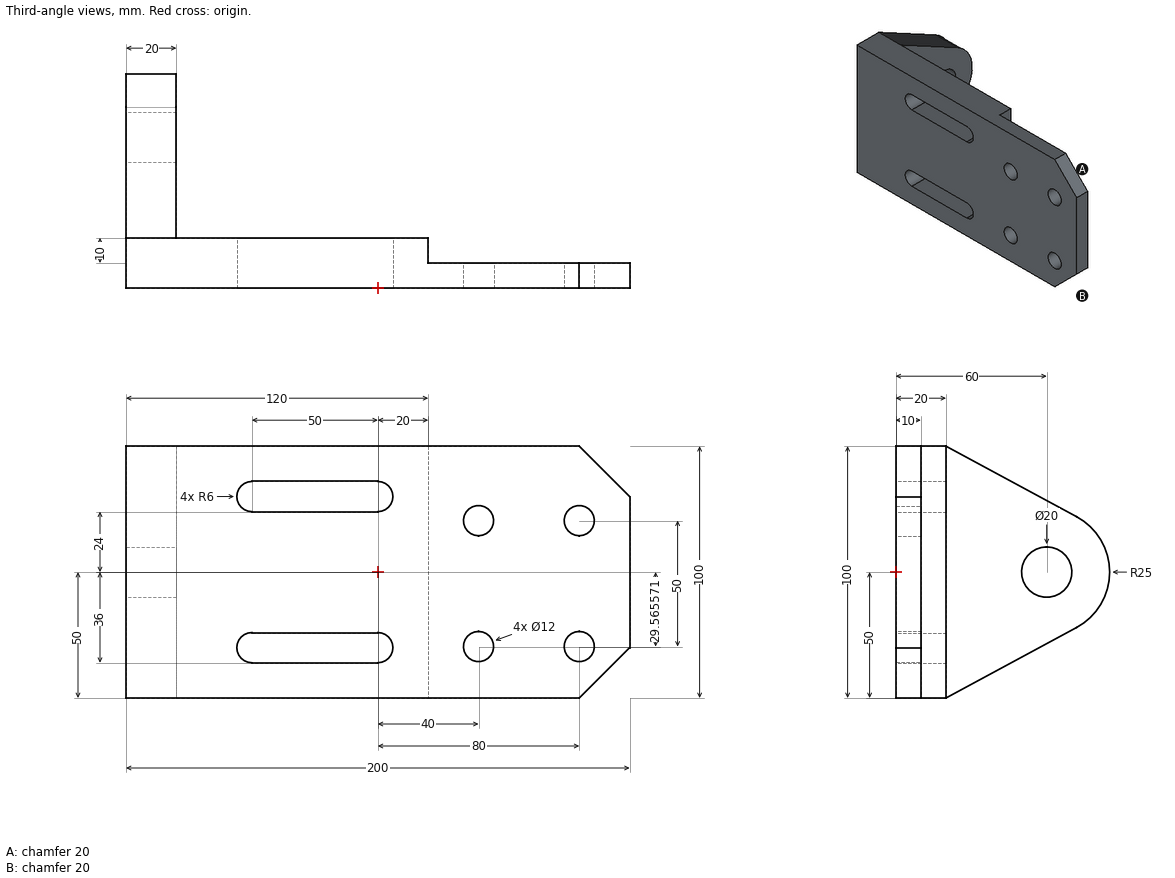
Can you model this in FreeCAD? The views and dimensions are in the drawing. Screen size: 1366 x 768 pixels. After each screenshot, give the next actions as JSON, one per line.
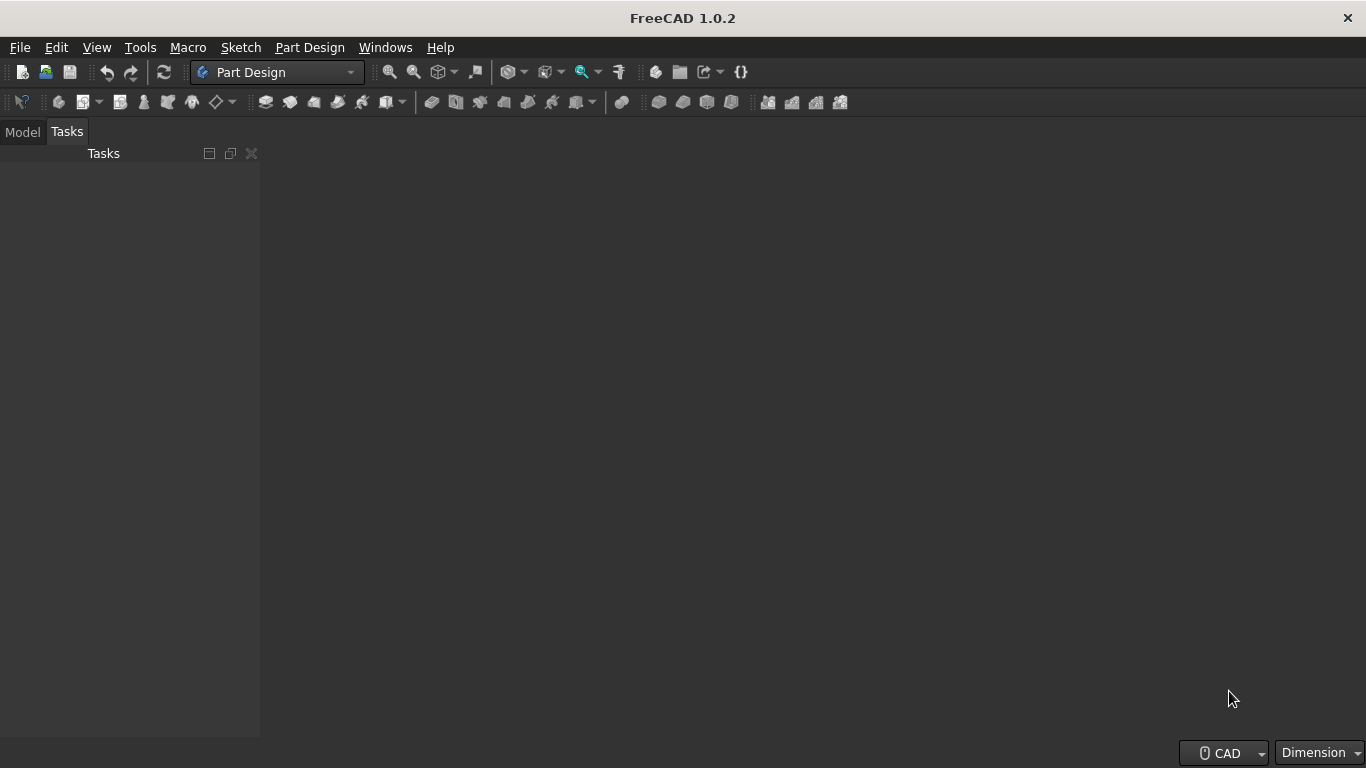
{"action": "left_click", "coordinate": [22, 72]}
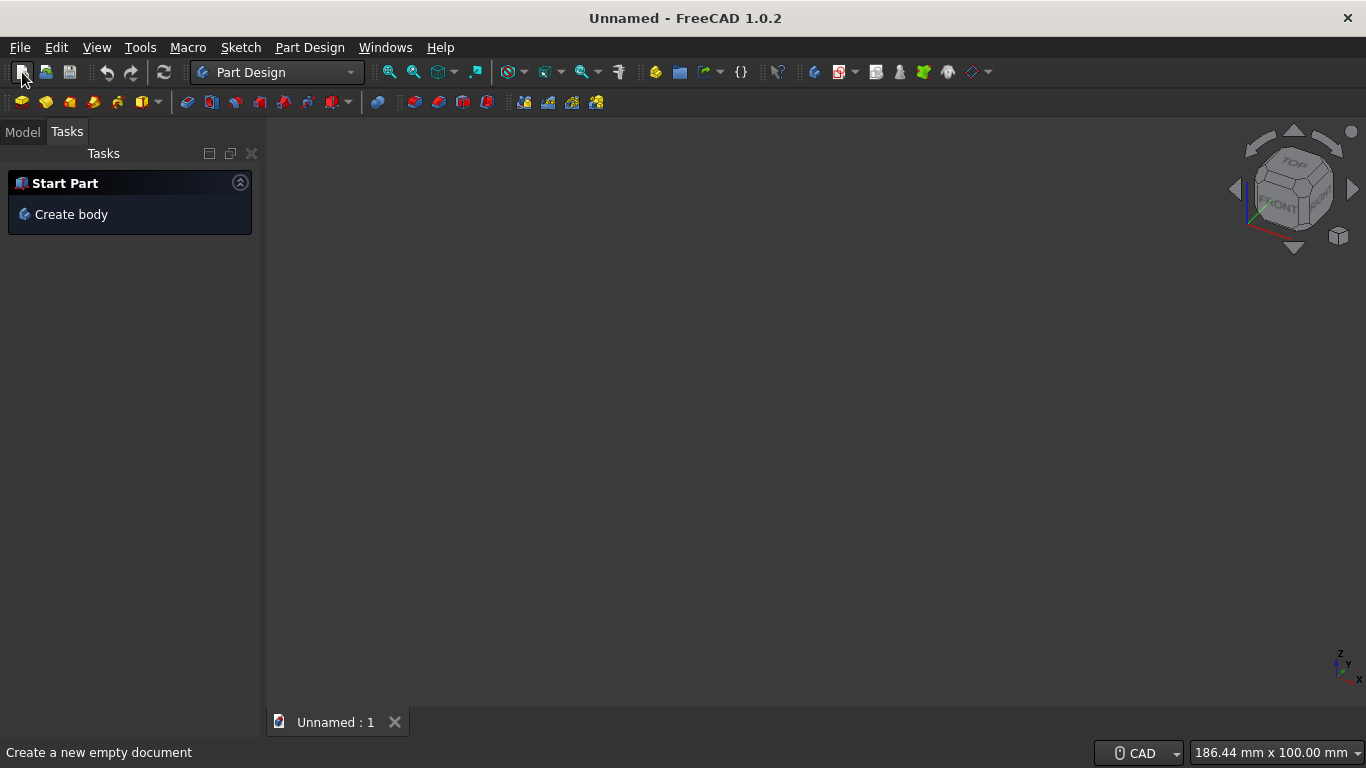
{"action": "left_click", "coordinate": [840, 72]}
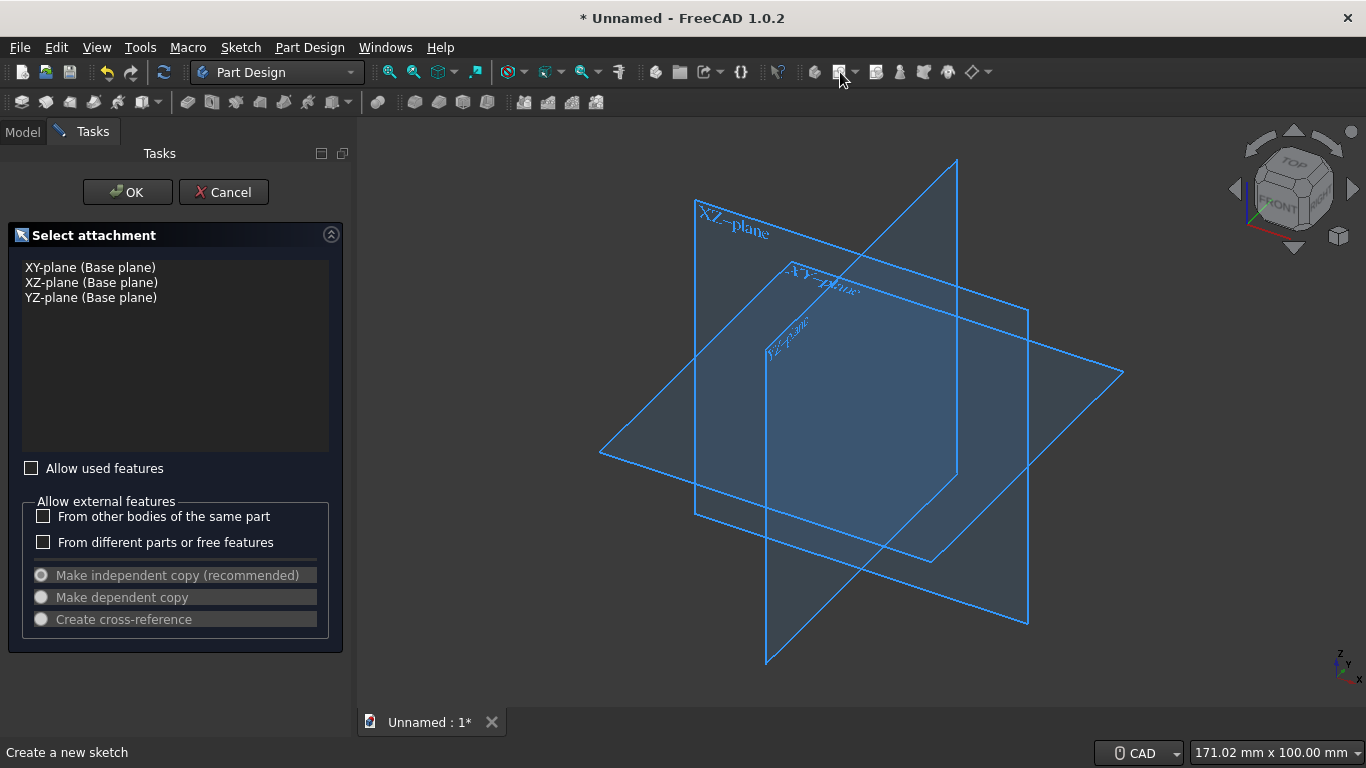
{"action": "left_click", "coordinate": [82, 282]}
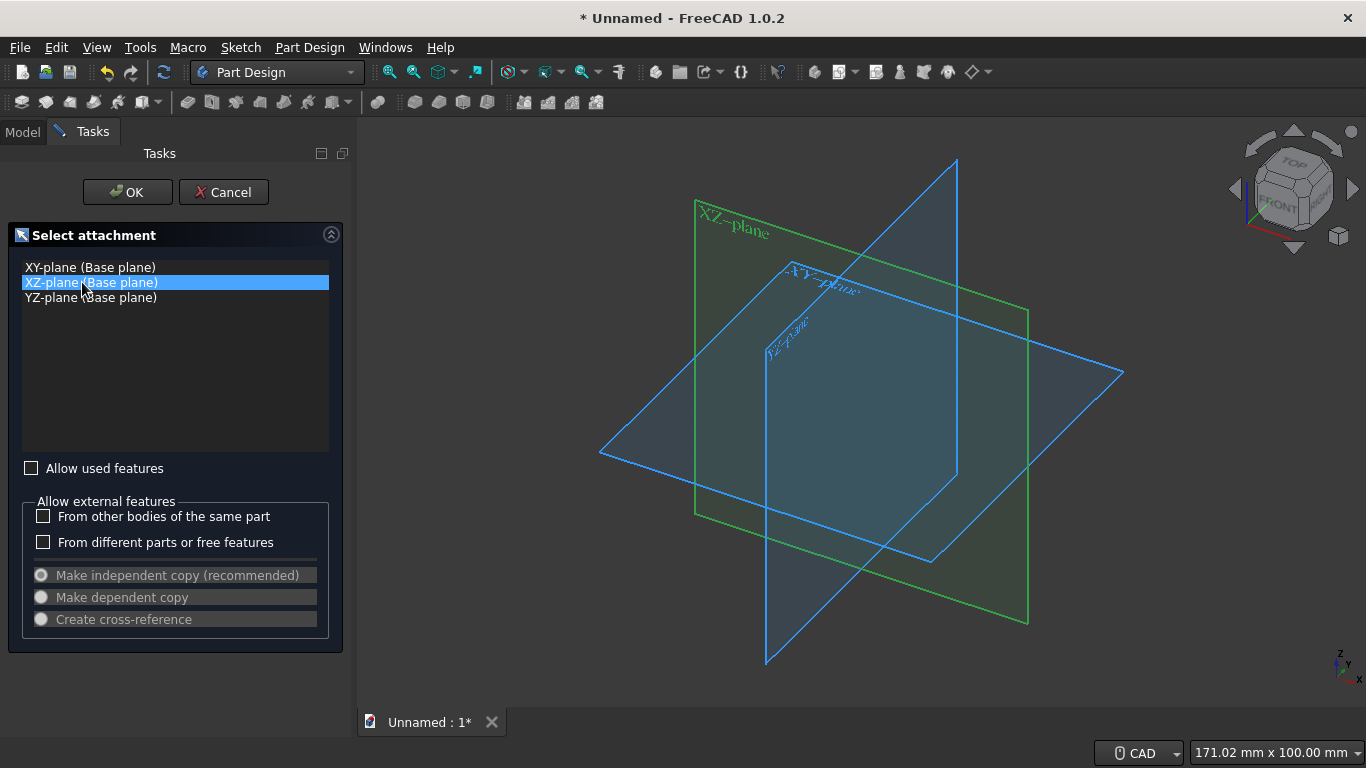
{"action": "left_click", "coordinate": [128, 192]}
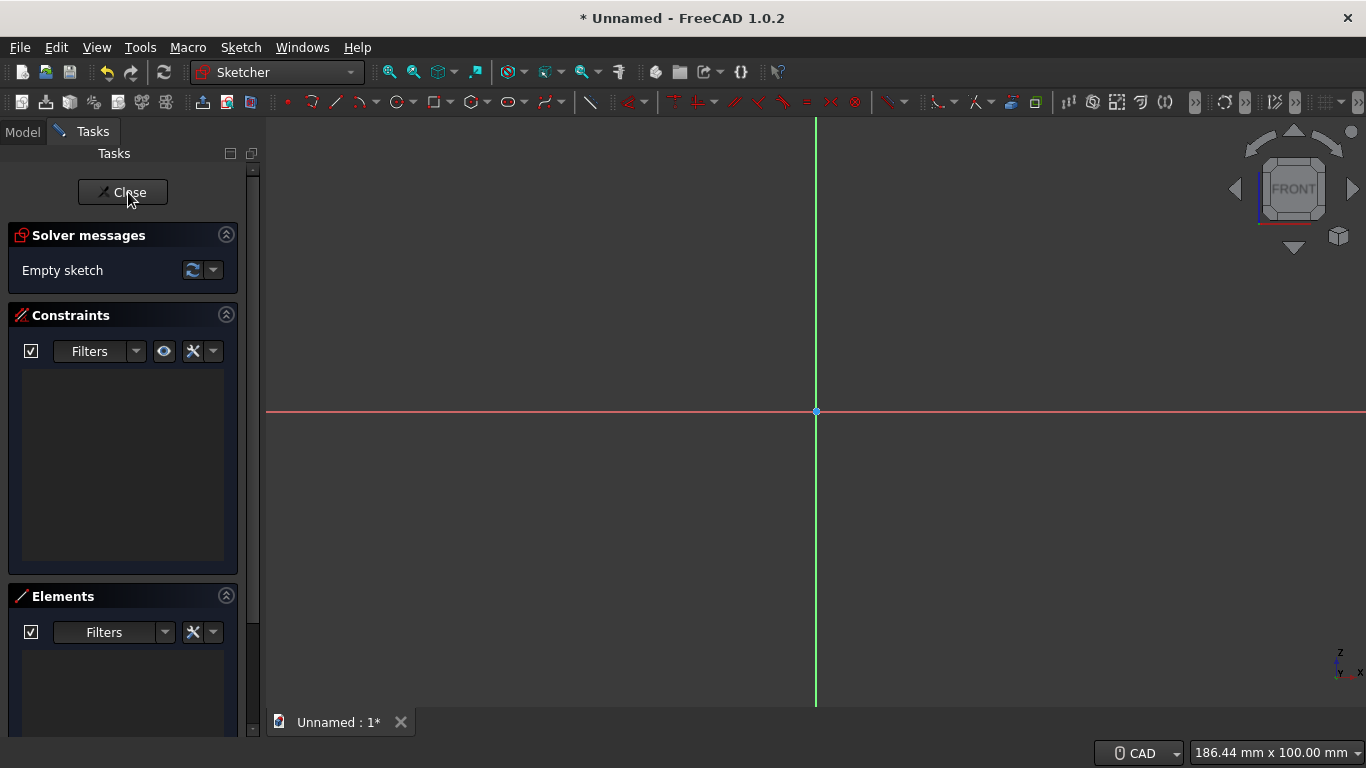
{"action": "scroll", "coordinate": [664, 412], "scroll_direction": "down", "scroll_amount": 3}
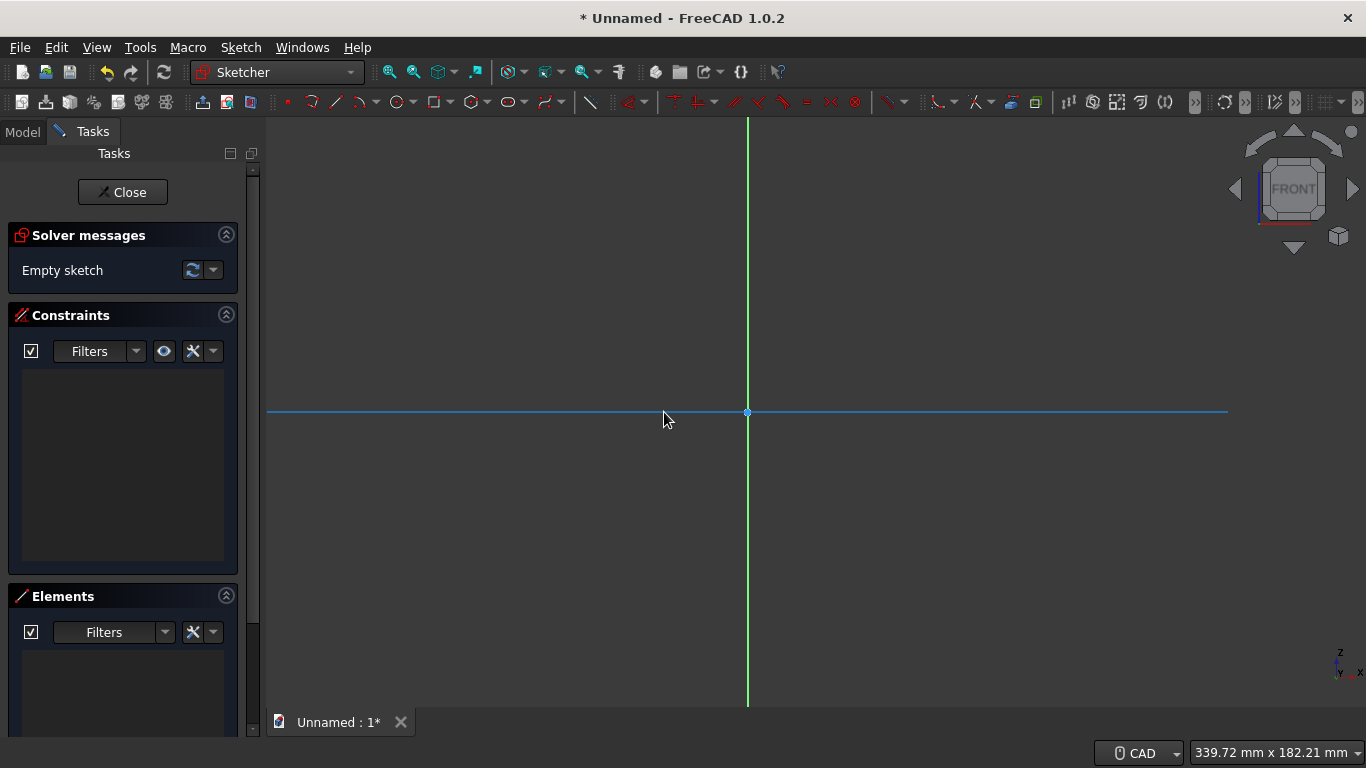
{"action": "key", "text": "g v"}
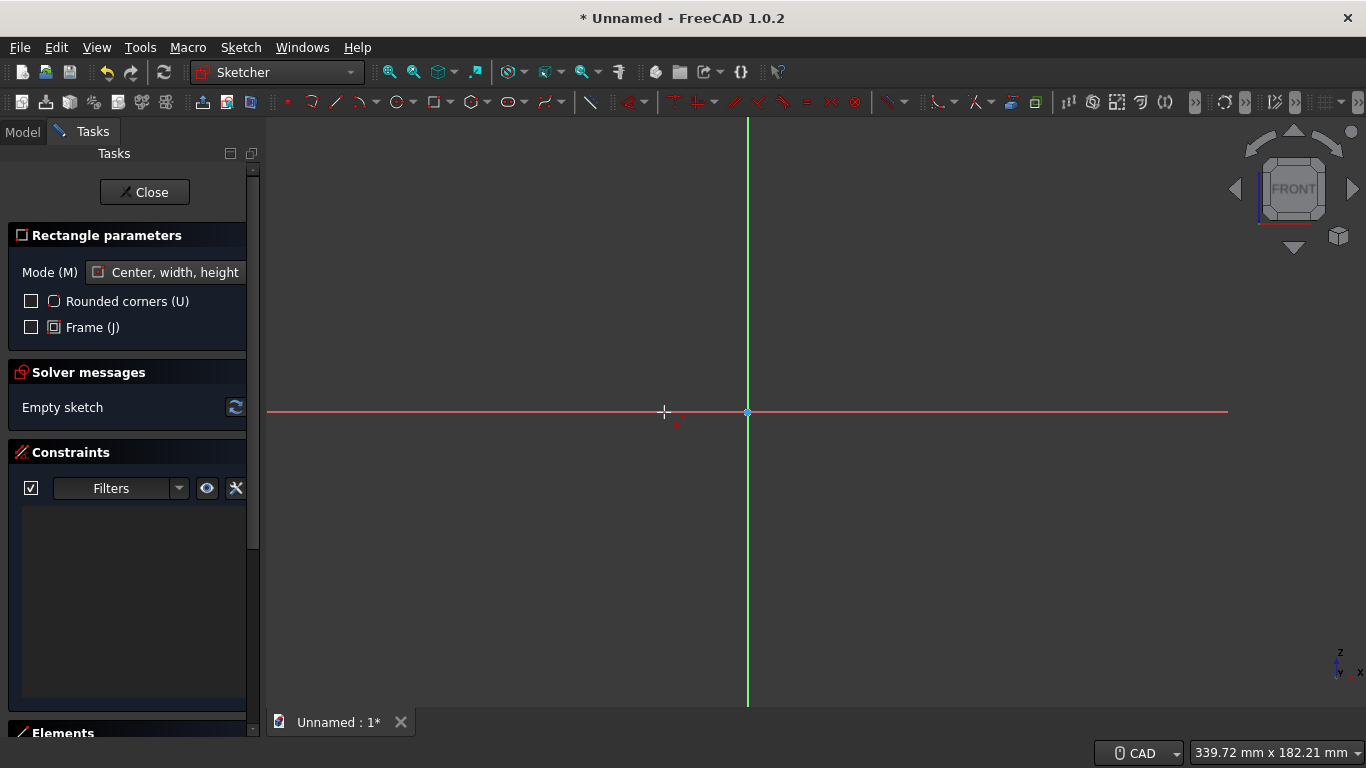
{"action": "left_click", "coordinate": [748, 412]}
{"action": "mouse_move", "coordinate": [1071, 250]}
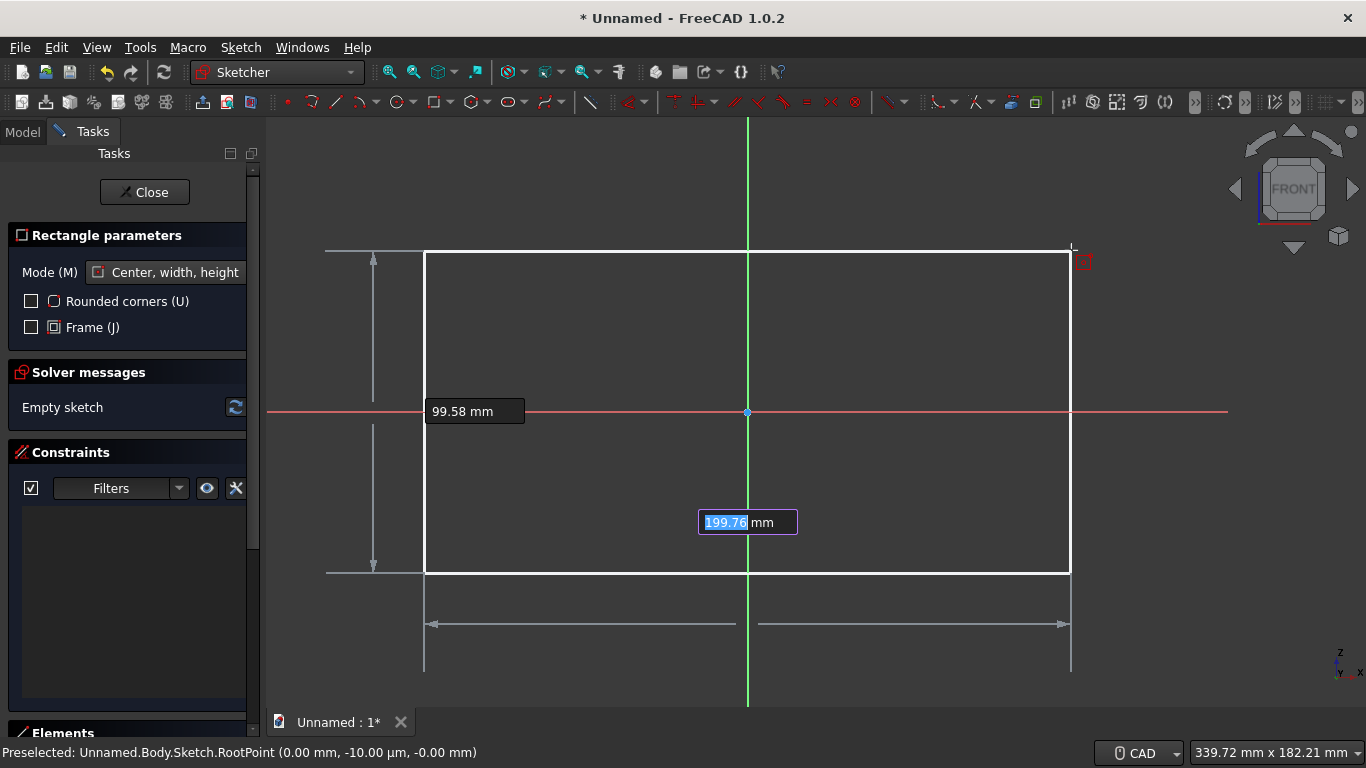
{"action": "type", "text": "200"}
{"action": "key", "text": "Tab"}
{"action": "type", "text": "100"}
{"action": "key", "text": "Return"}
{"action": "key", "text": "Escape"}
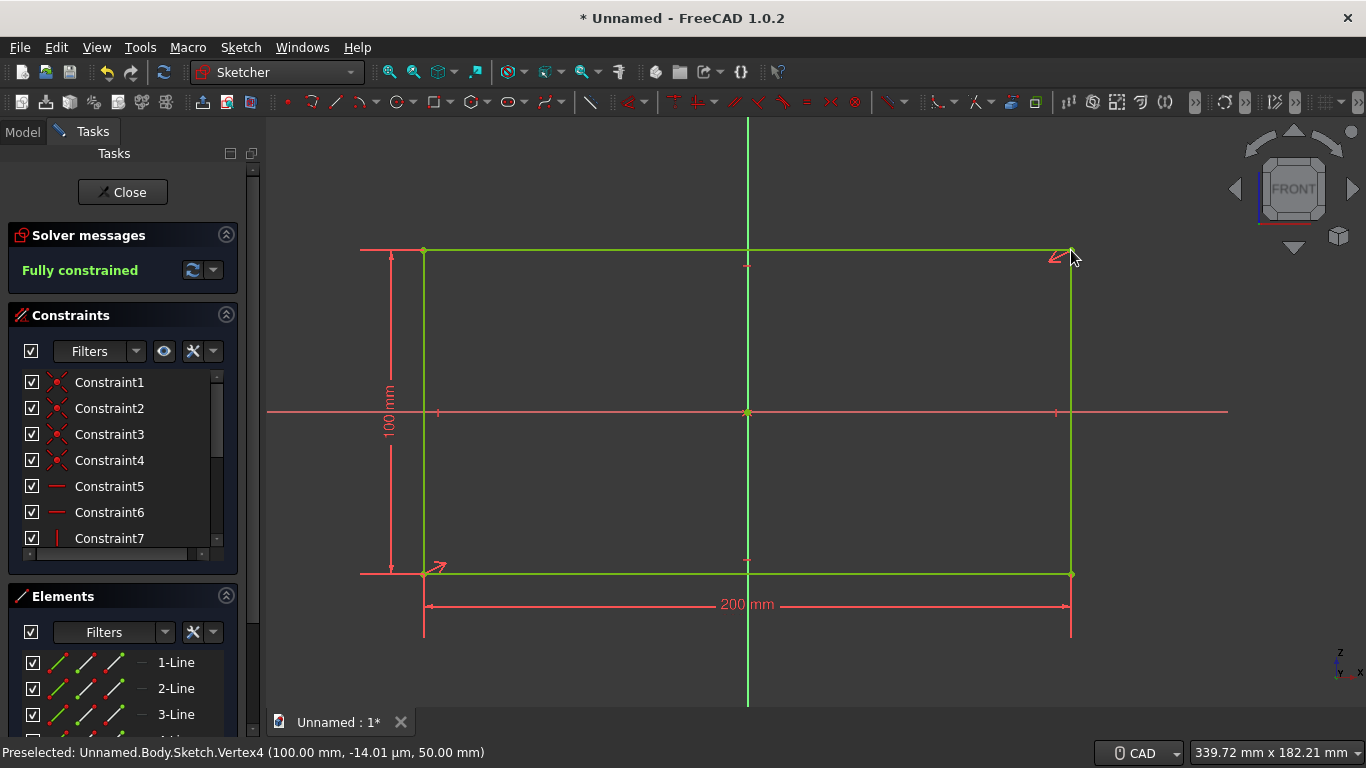
{"action": "left_click", "coordinate": [123, 192]}